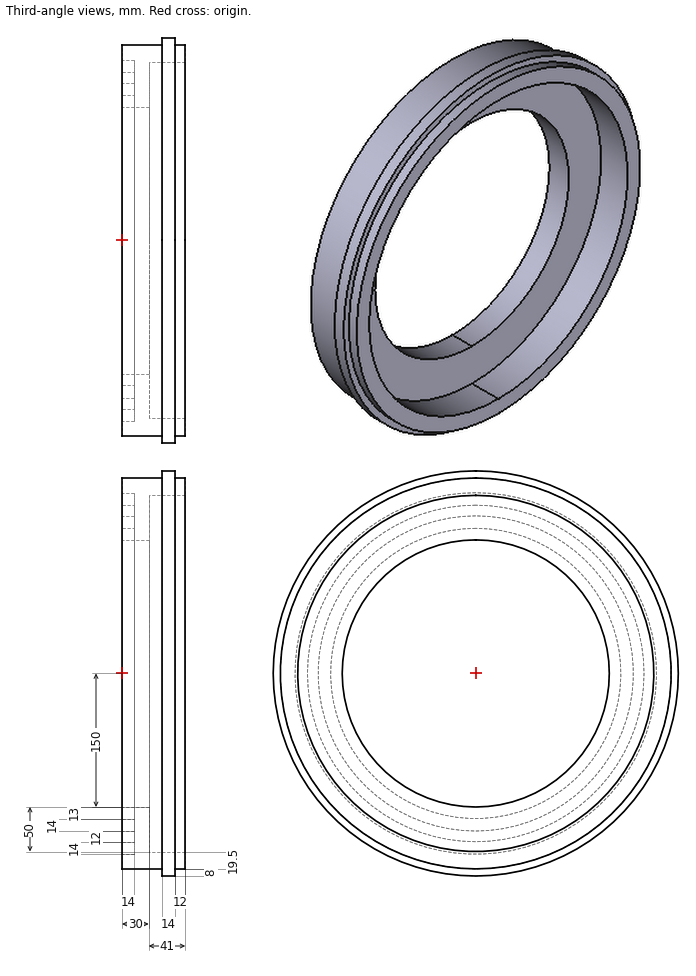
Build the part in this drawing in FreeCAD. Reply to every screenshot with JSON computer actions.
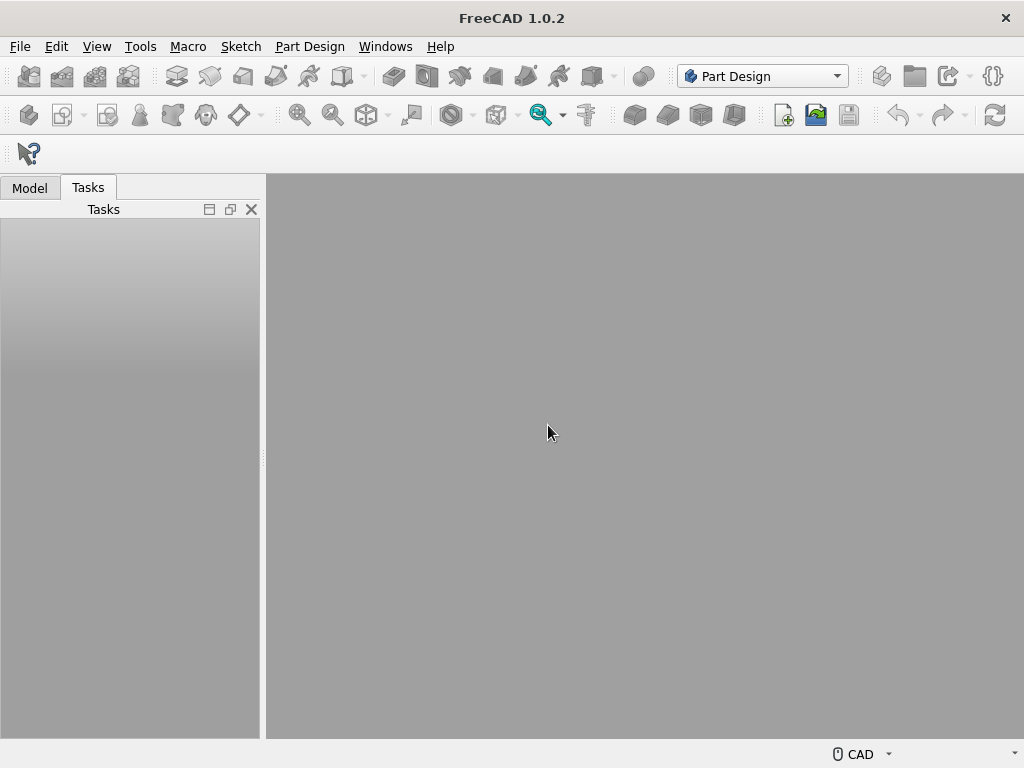
{"action": "left_click", "coordinate": [783, 116]}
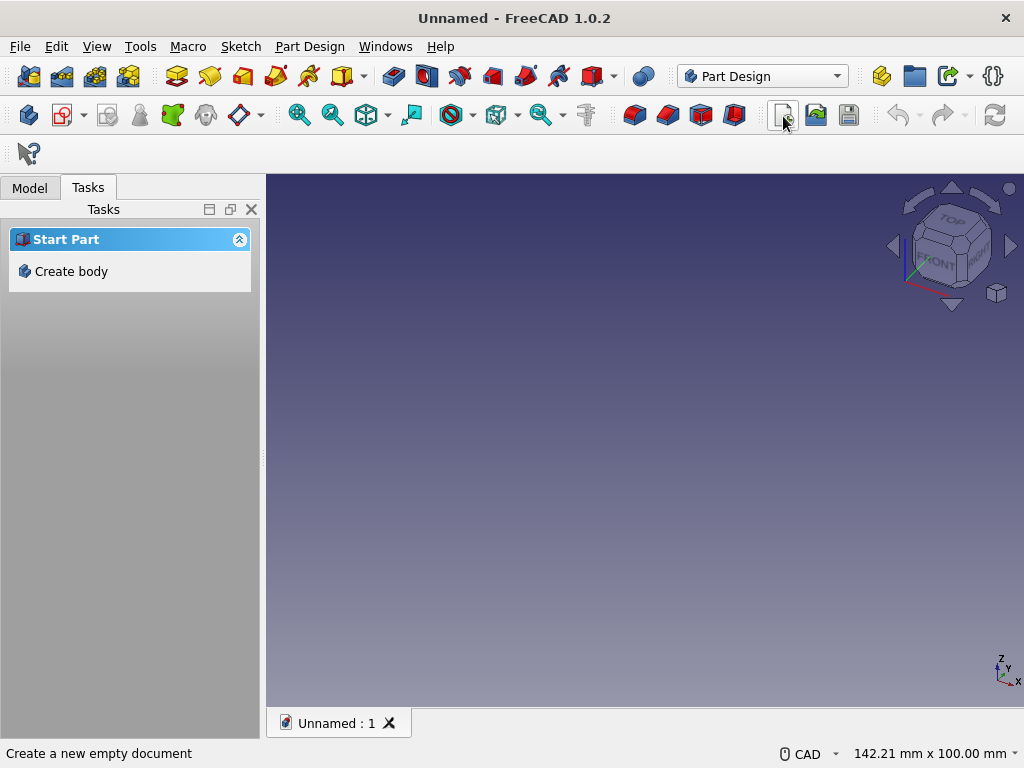
{"action": "left_click", "coordinate": [62, 116]}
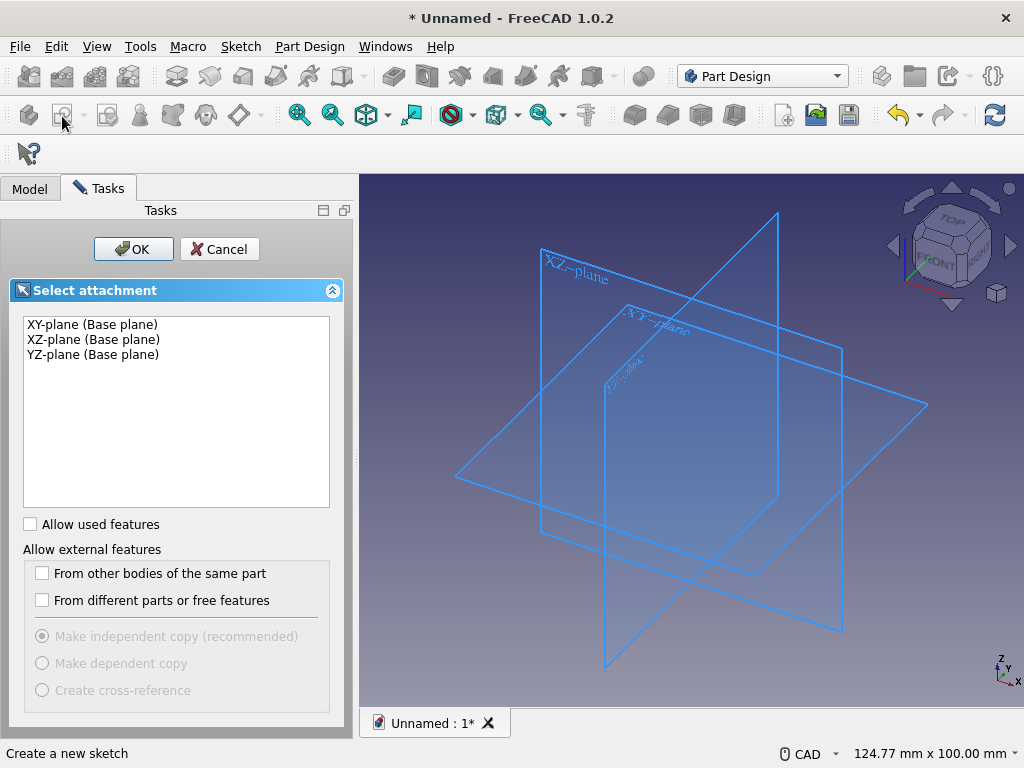
{"action": "left_click", "coordinate": [84, 340]}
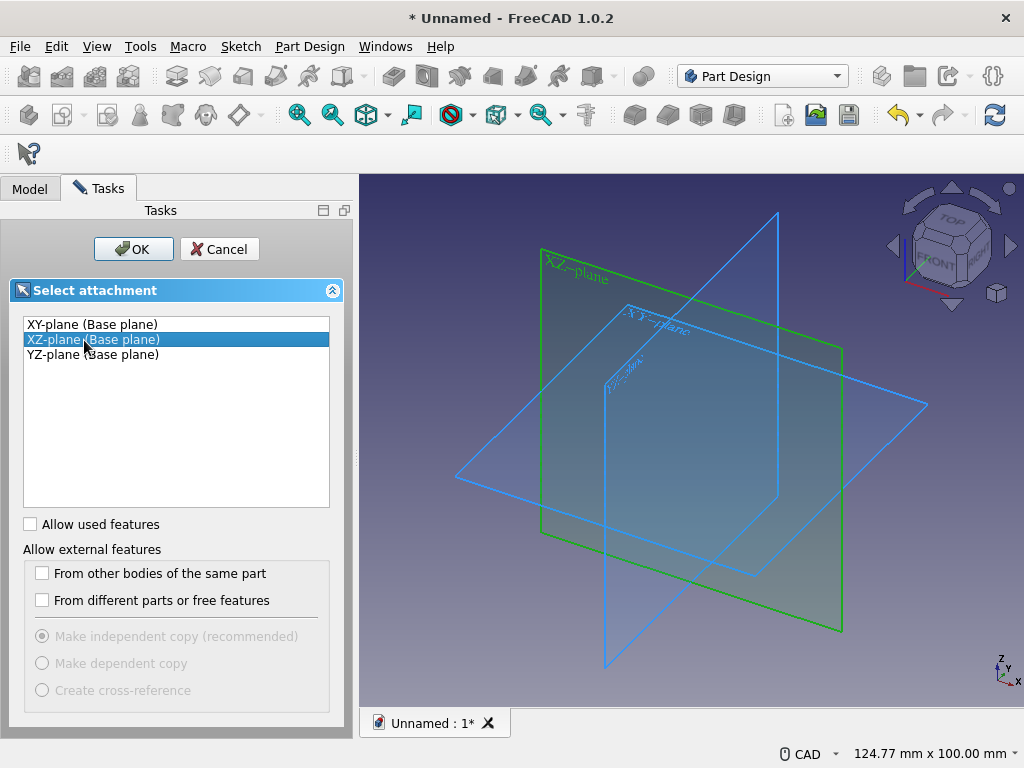
{"action": "left_click", "coordinate": [134, 249]}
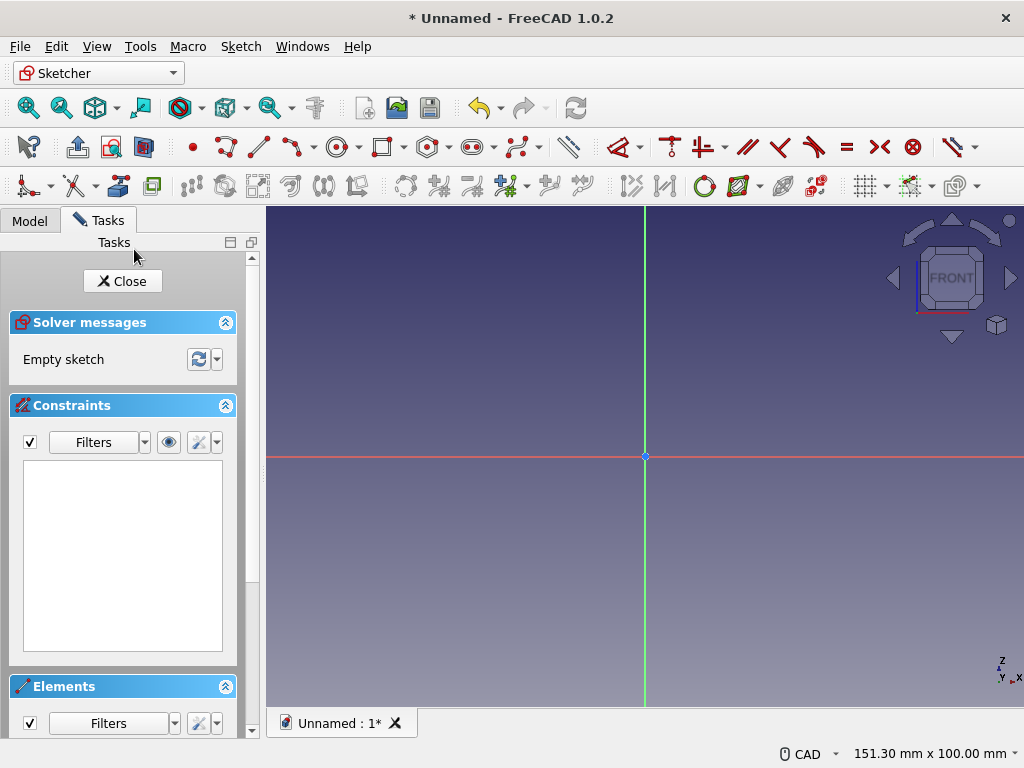
{"action": "scroll", "coordinate": [576, 456], "scroll_direction": "down", "scroll_amount": 5}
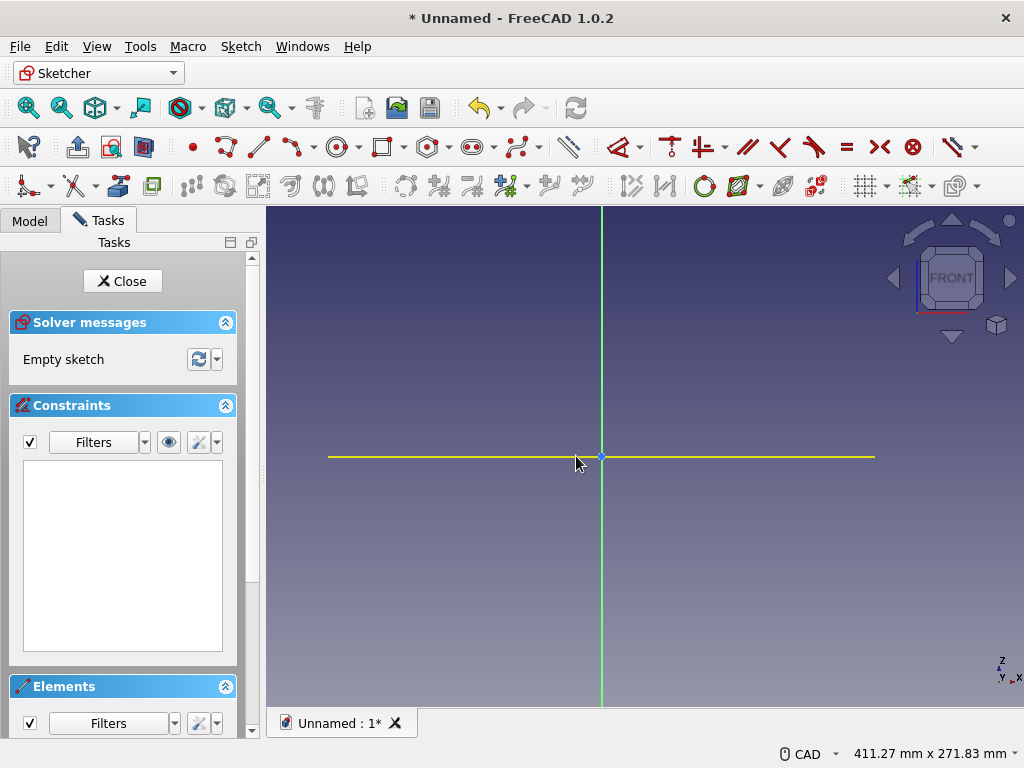
{"action": "scroll", "coordinate": [576, 456], "scroll_direction": "down", "scroll_amount": 5}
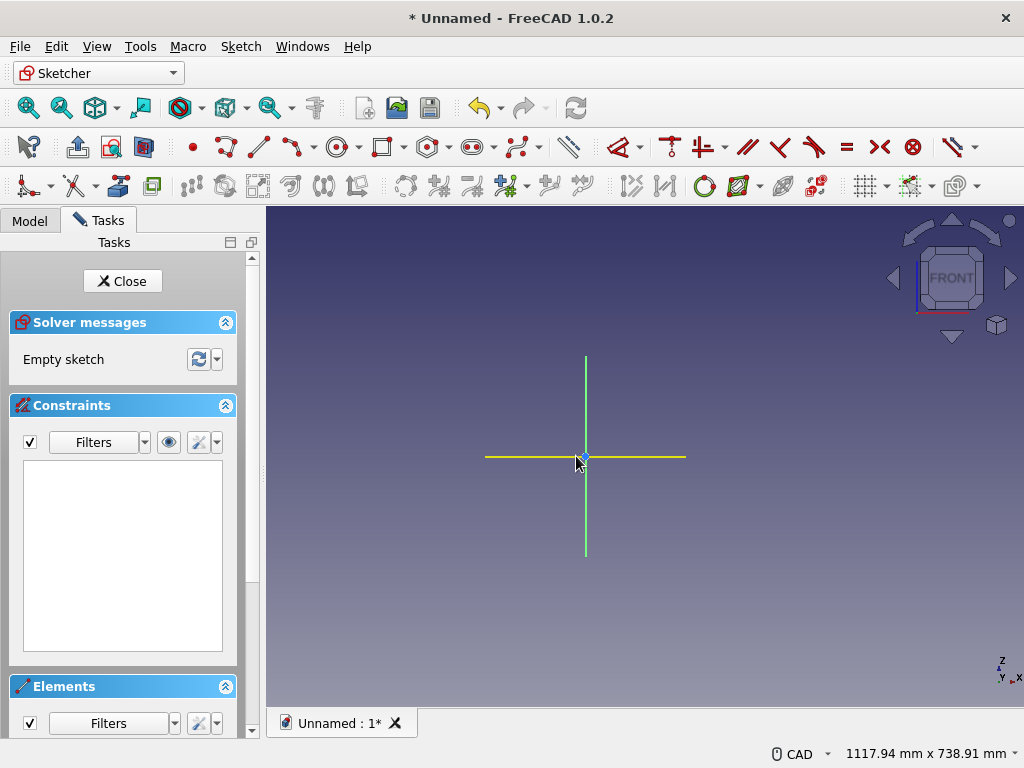
{"action": "scroll", "coordinate": [616, 610], "scroll_direction": "up", "scroll_amount": 9}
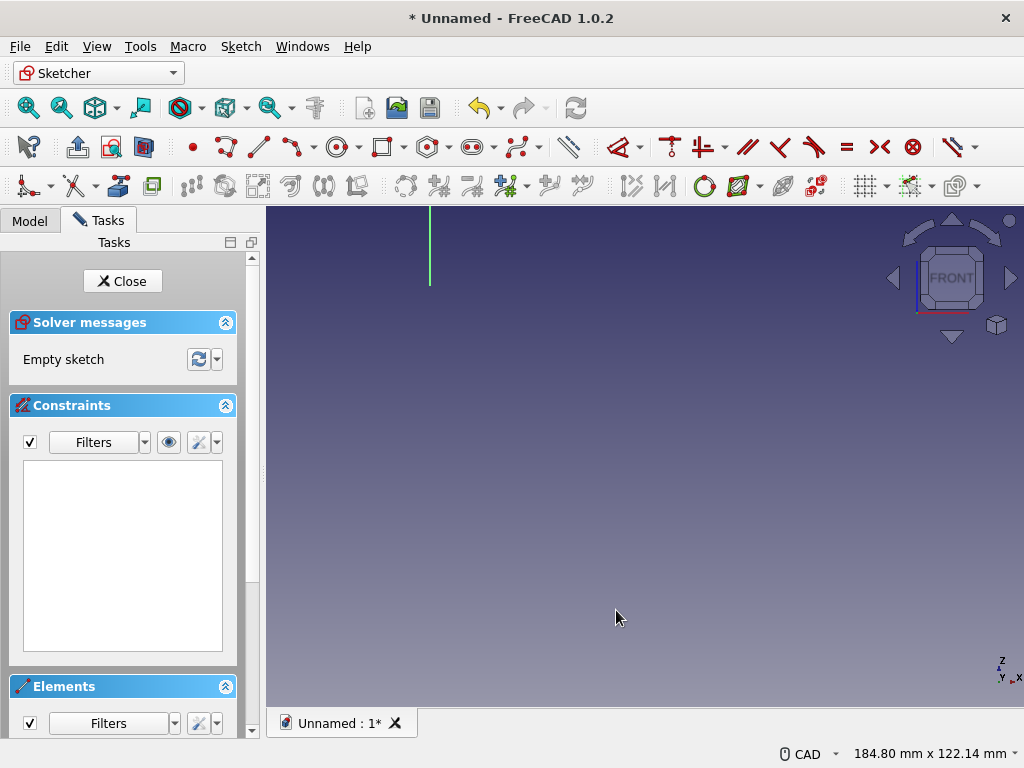
{"action": "left_click", "coordinate": [226, 148]}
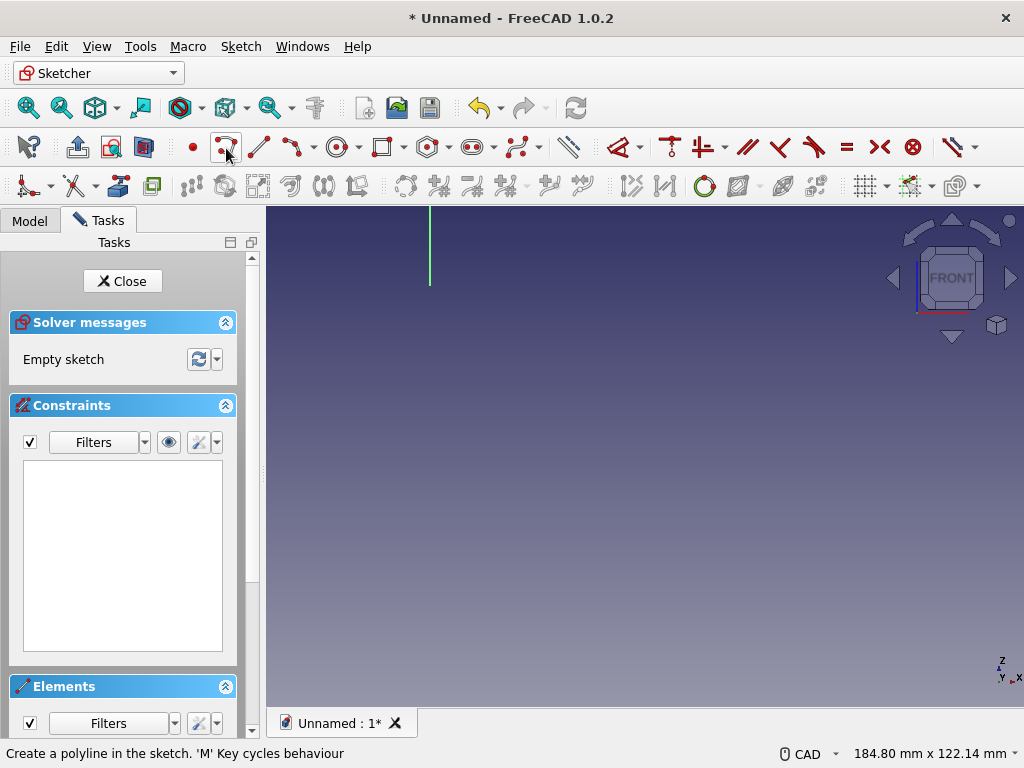
{"action": "left_click", "coordinate": [430, 293]}
{"action": "left_click", "coordinate": [553, 293]}
{"action": "left_click", "coordinate": [553, 498]}
{"action": "left_click", "coordinate": [722, 498]}
{"action": "left_click", "coordinate": [722, 578]}
{"action": "left_click", "coordinate": [672, 578]}
{"action": "left_click", "coordinate": [672, 610]}
{"action": "left_click", "coordinate": [615, 610]}
{"action": "left_click", "coordinate": [615, 578]}
{"action": "left_click", "coordinate": [430, 578]}
{"action": "left_click", "coordinate": [439, 510]}
{"action": "left_click", "coordinate": [488, 510]}
{"action": "left_click", "coordinate": [488, 453]}
{"action": "left_click", "coordinate": [430, 453]}
{"action": "left_click", "coordinate": [439, 403]}
{"action": "left_click", "coordinate": [488, 403]}
{"action": "left_click", "coordinate": [488, 346]}
{"action": "left_click", "coordinate": [439, 346]}
{"action": "left_click", "coordinate": [430, 294]}
{"action": "key", "text": "Escape"}
{"action": "key", "text": "Escape"}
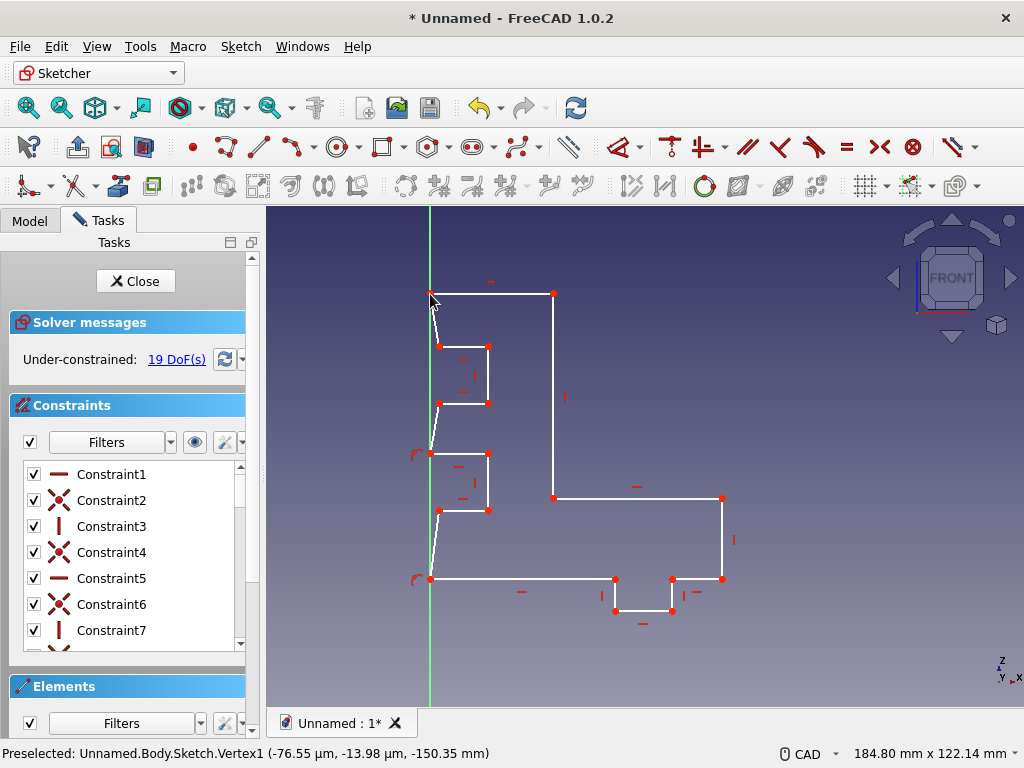
{"action": "left_click", "coordinate": [433, 559]}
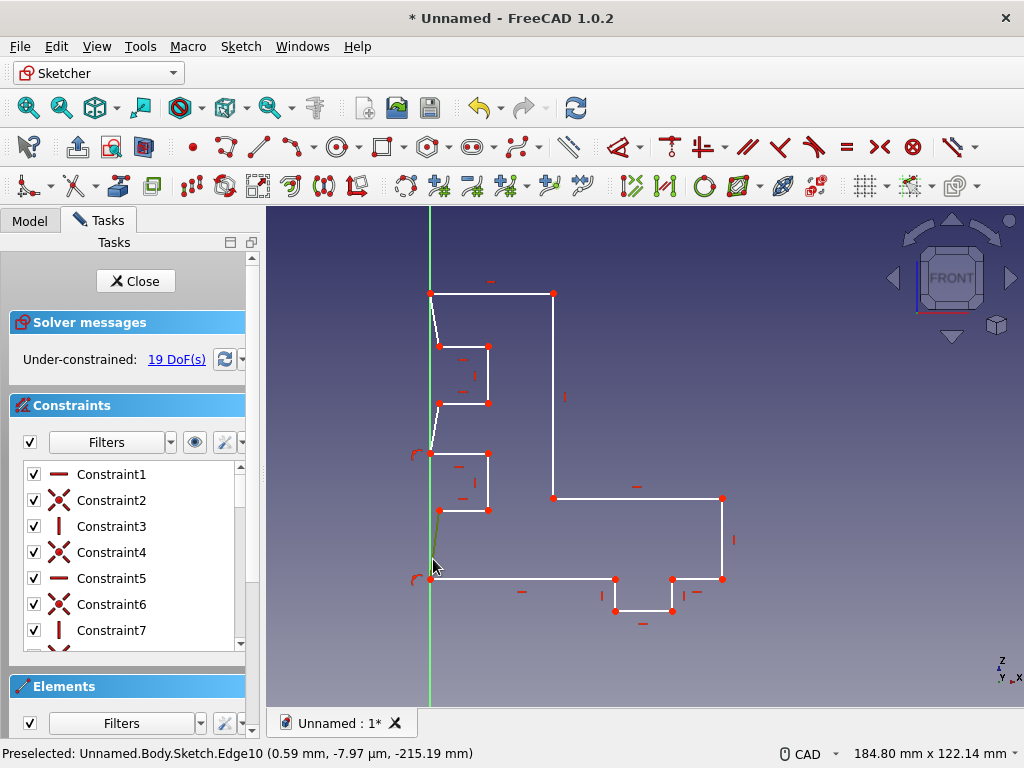
{"action": "key", "text": "v"}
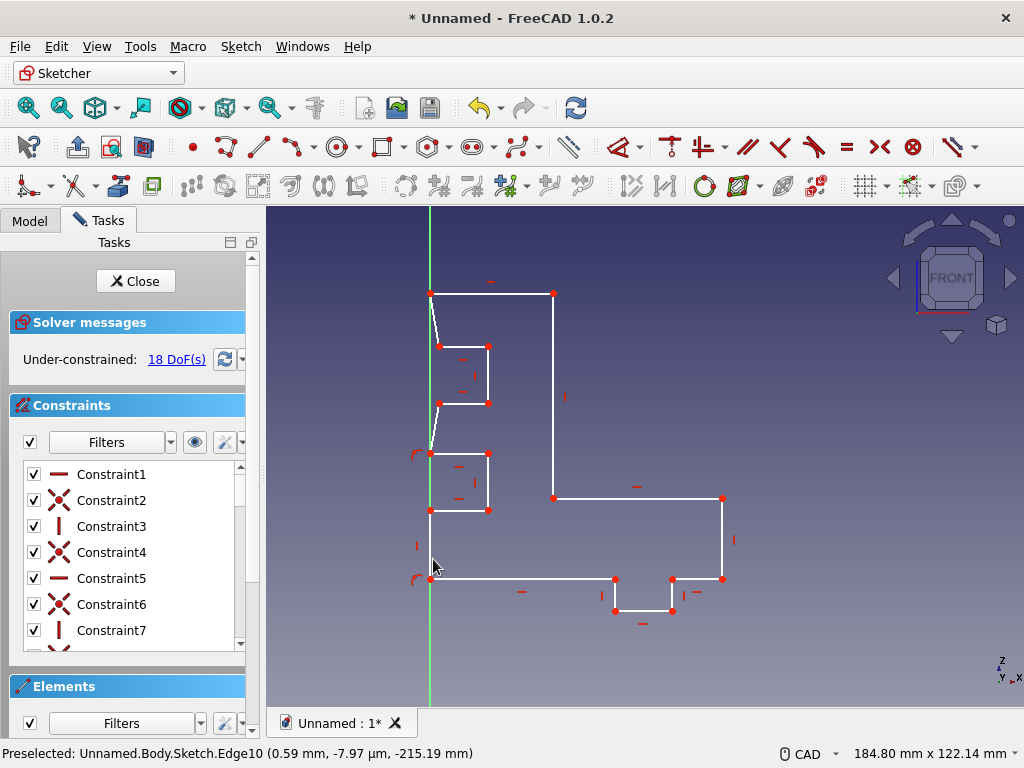
{"action": "left_click", "coordinate": [433, 439]}